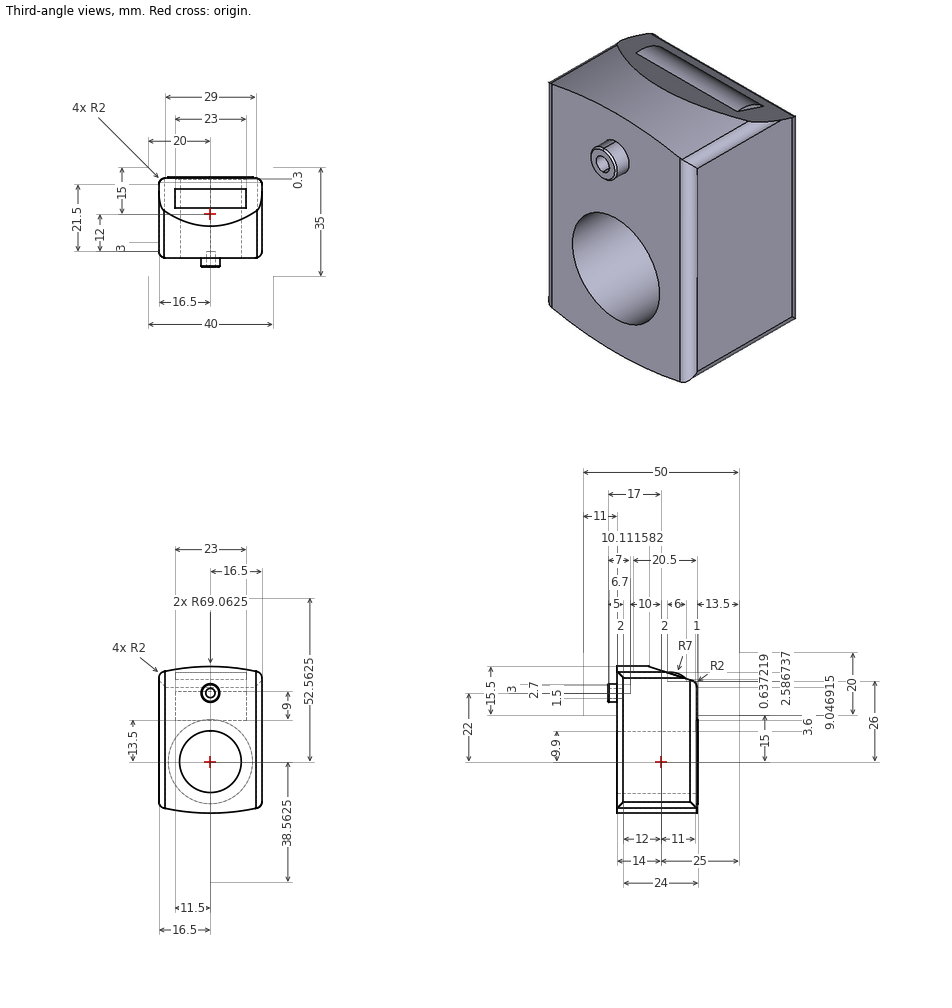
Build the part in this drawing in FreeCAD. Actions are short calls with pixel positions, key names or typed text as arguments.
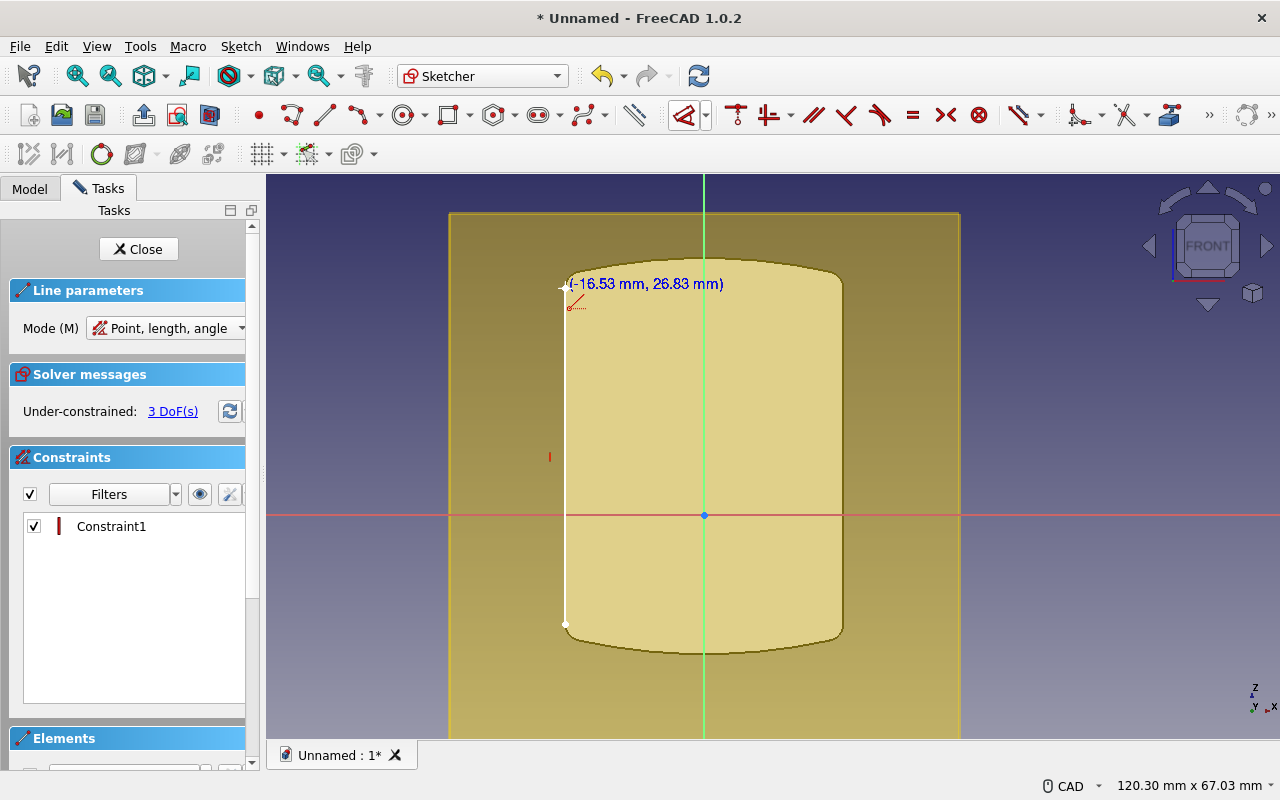
click(843, 288)
click(843, 624)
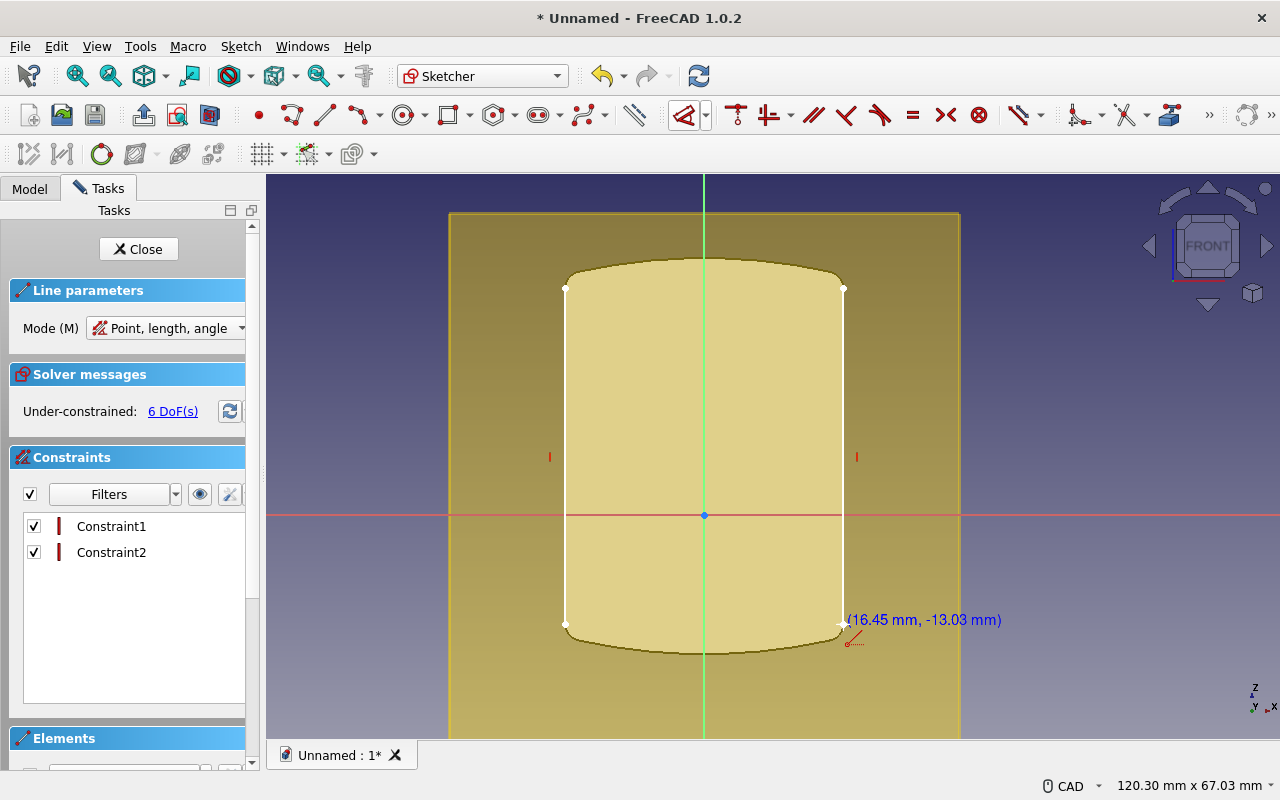
click(358, 116)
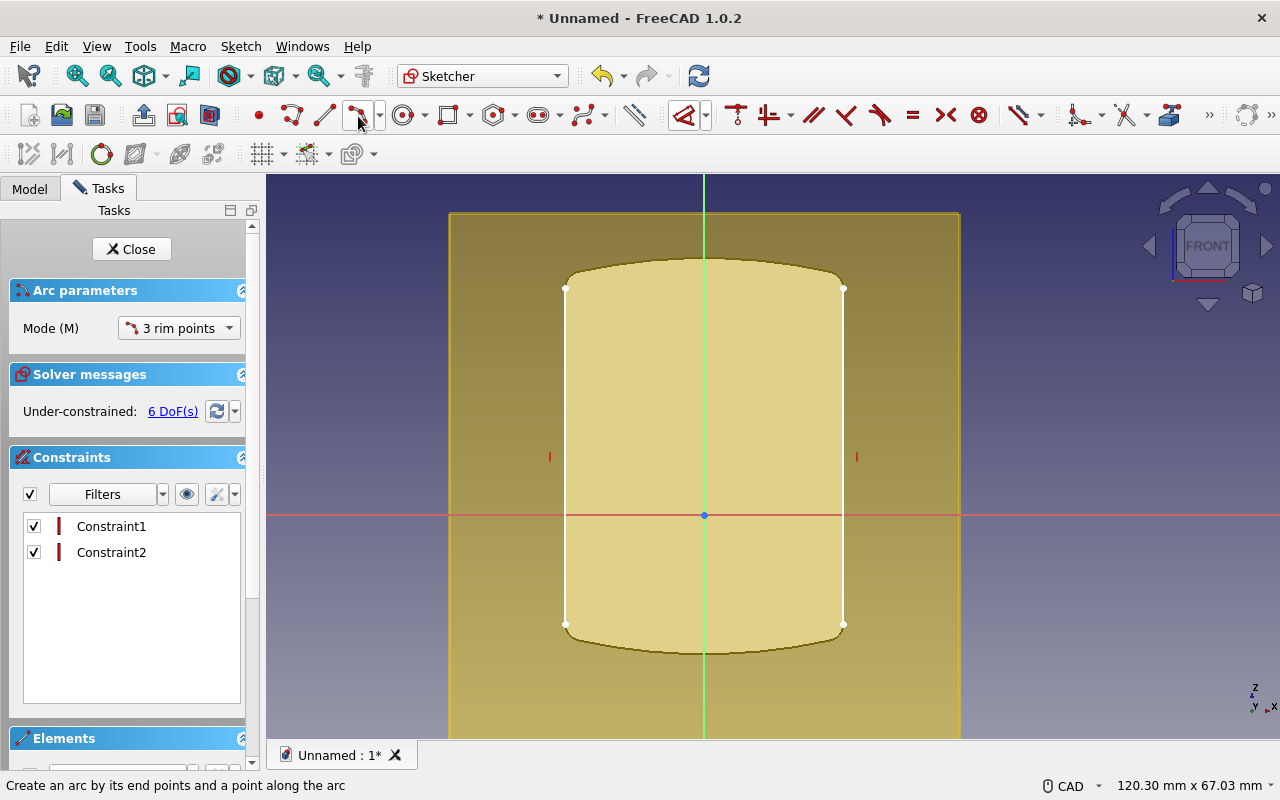
click(565, 289)
click(578, 272)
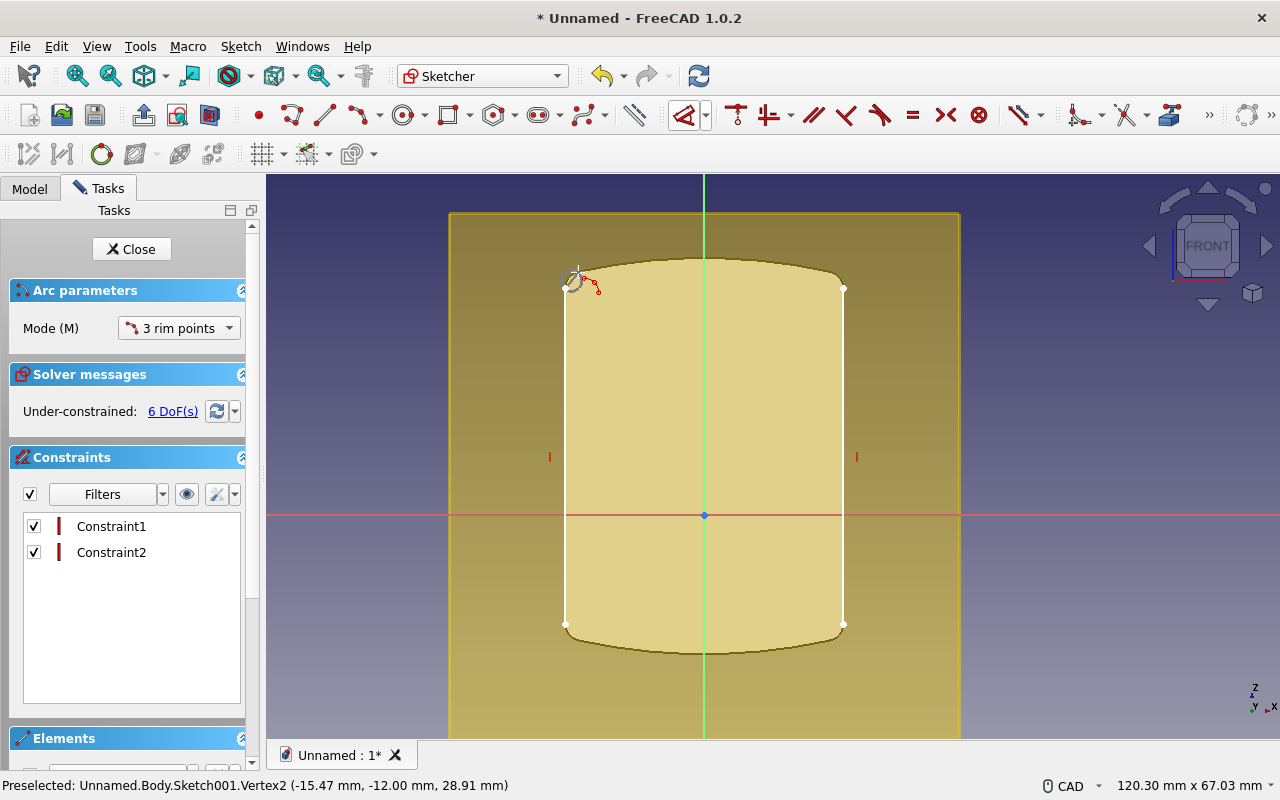
scroll(569, 278, up, 8)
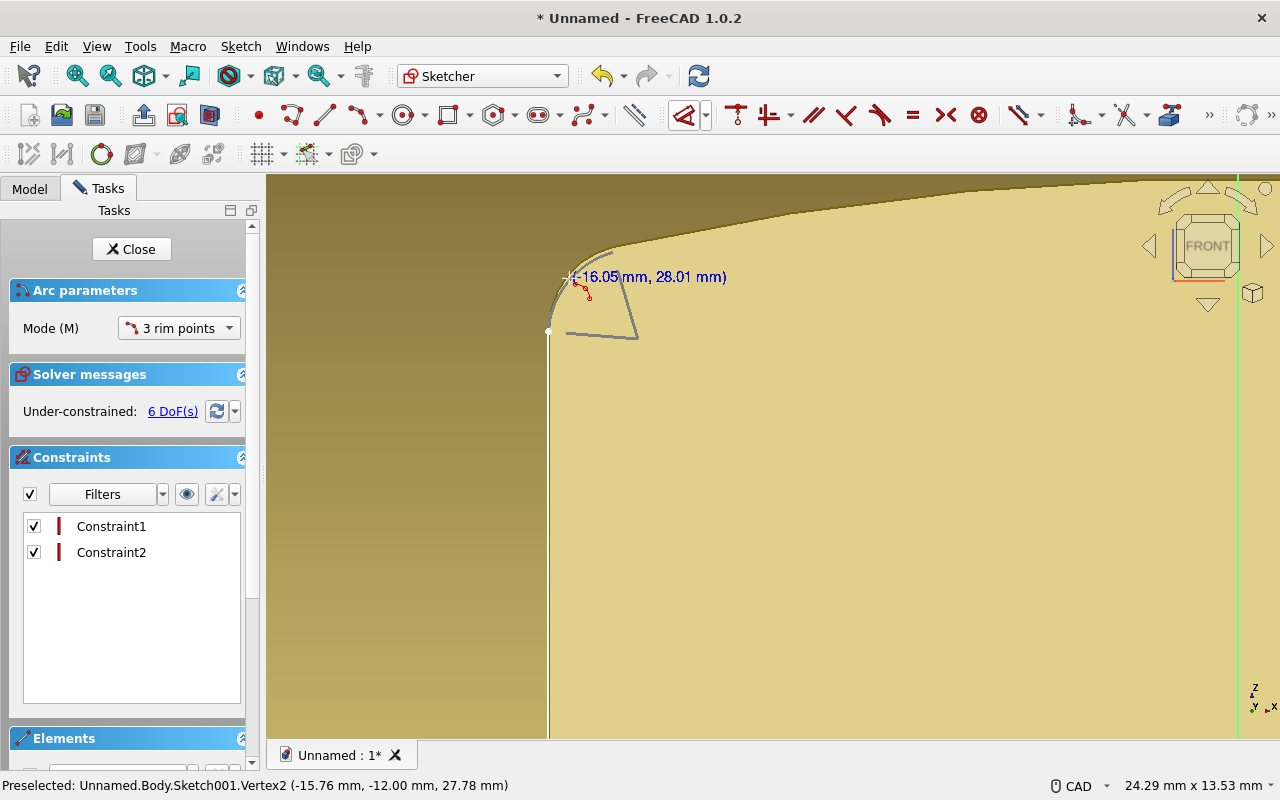
click(568, 276)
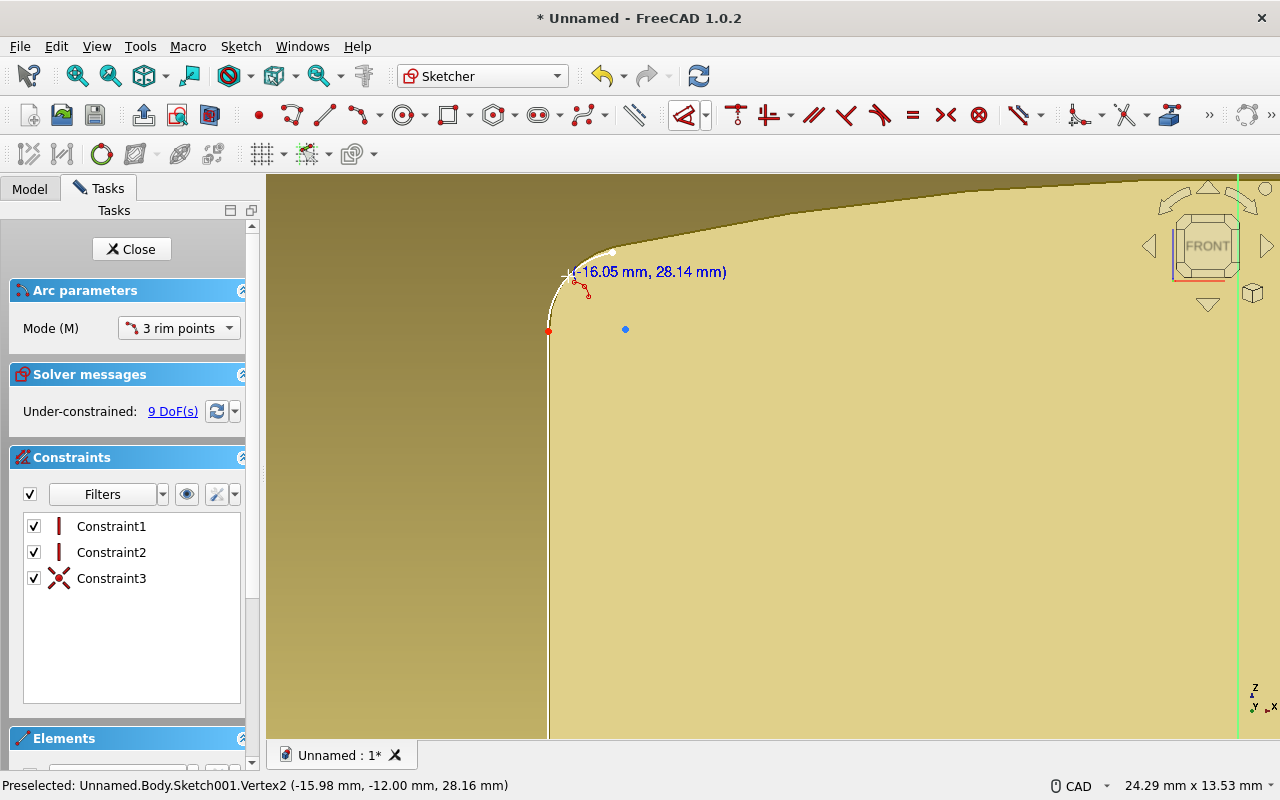
scroll(570, 279, down, 8)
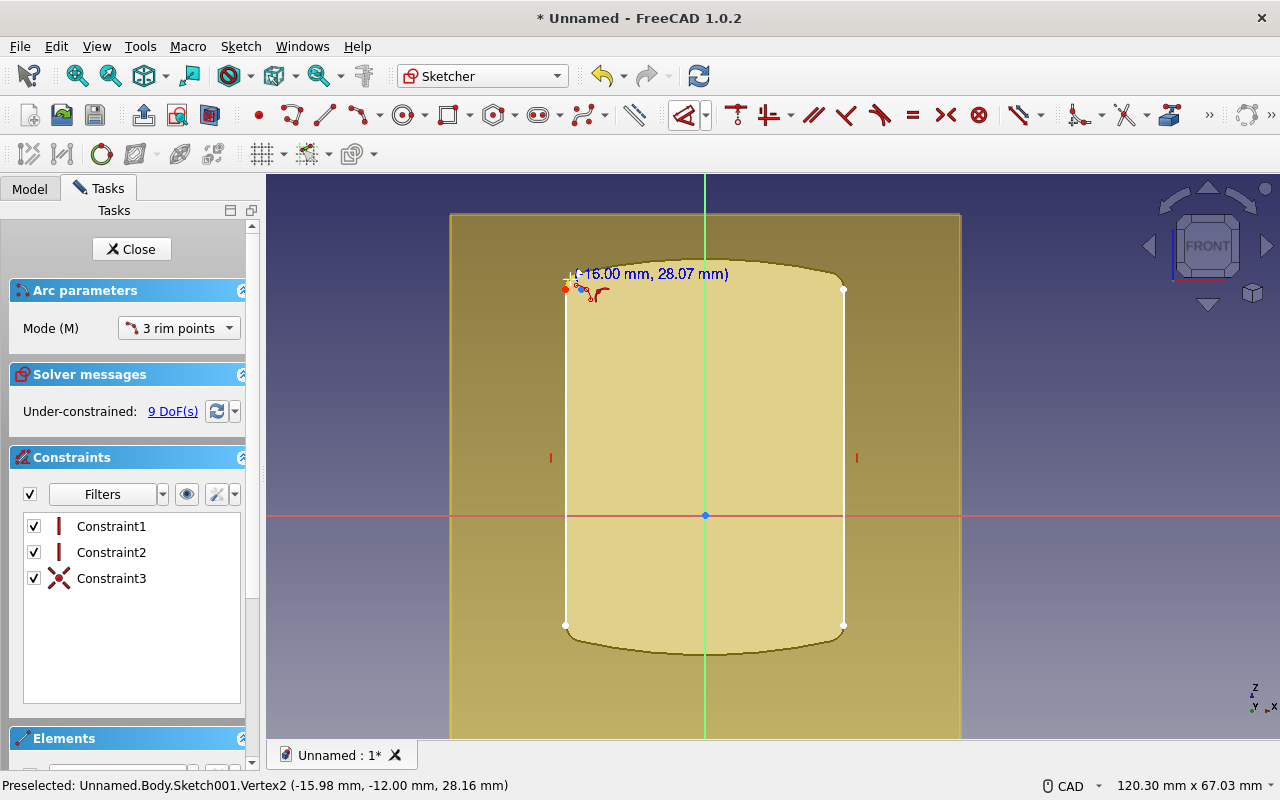
click(579, 274)
click(831, 273)
click(730, 259)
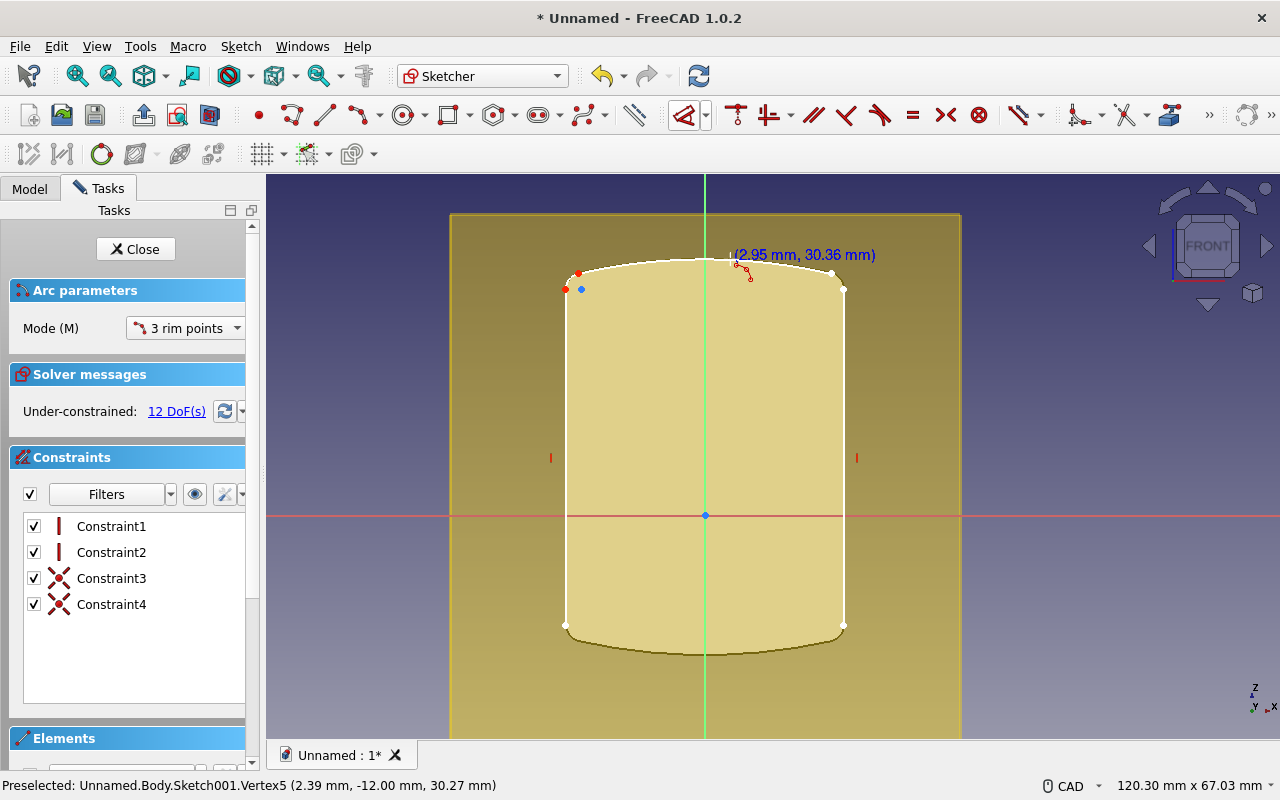
click(831, 274)
click(844, 290)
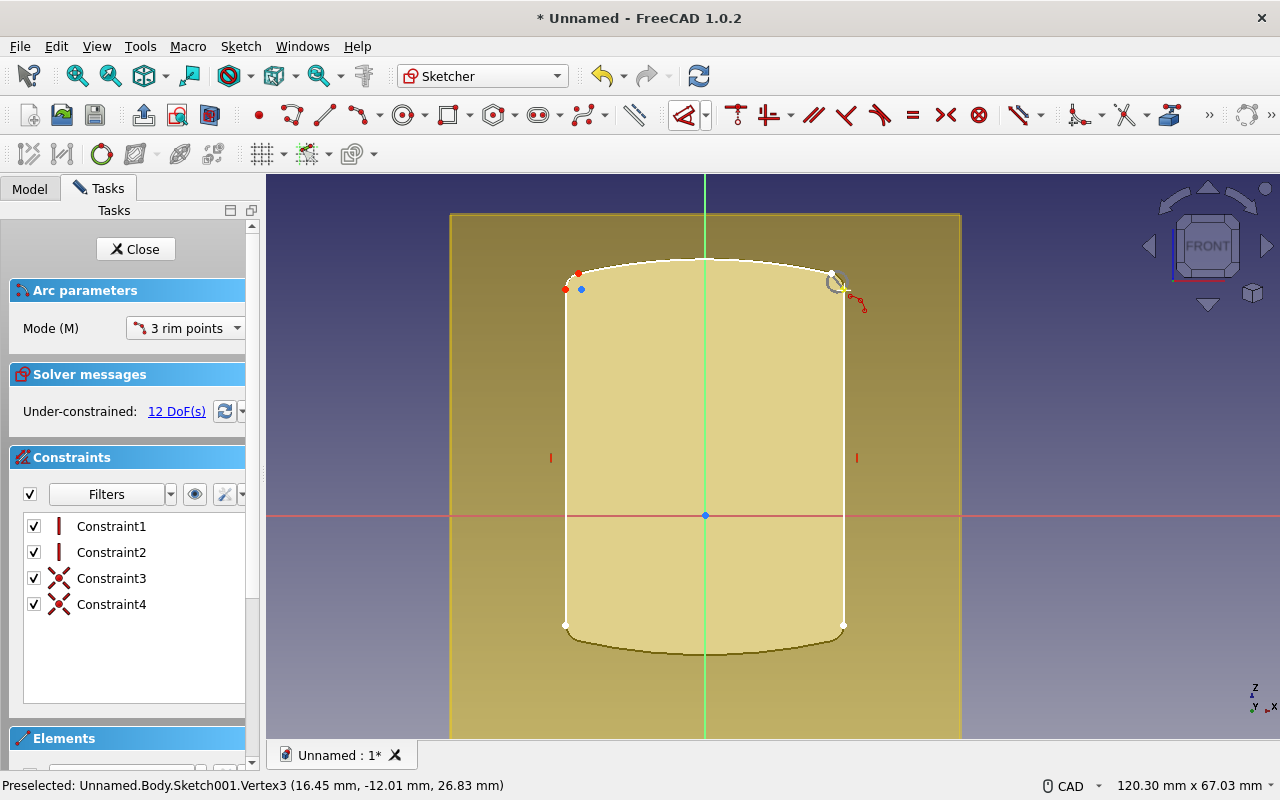
scroll(840, 279, up, 8)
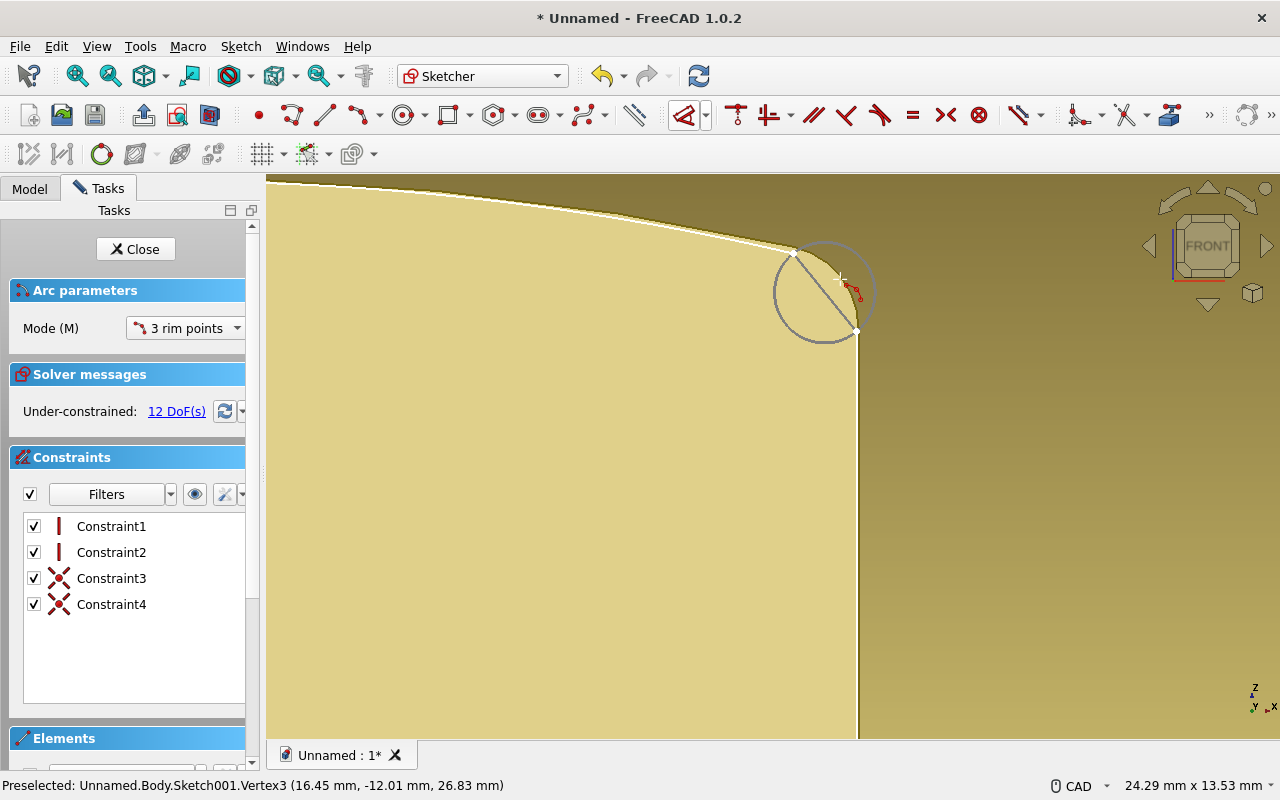
click(840, 276)